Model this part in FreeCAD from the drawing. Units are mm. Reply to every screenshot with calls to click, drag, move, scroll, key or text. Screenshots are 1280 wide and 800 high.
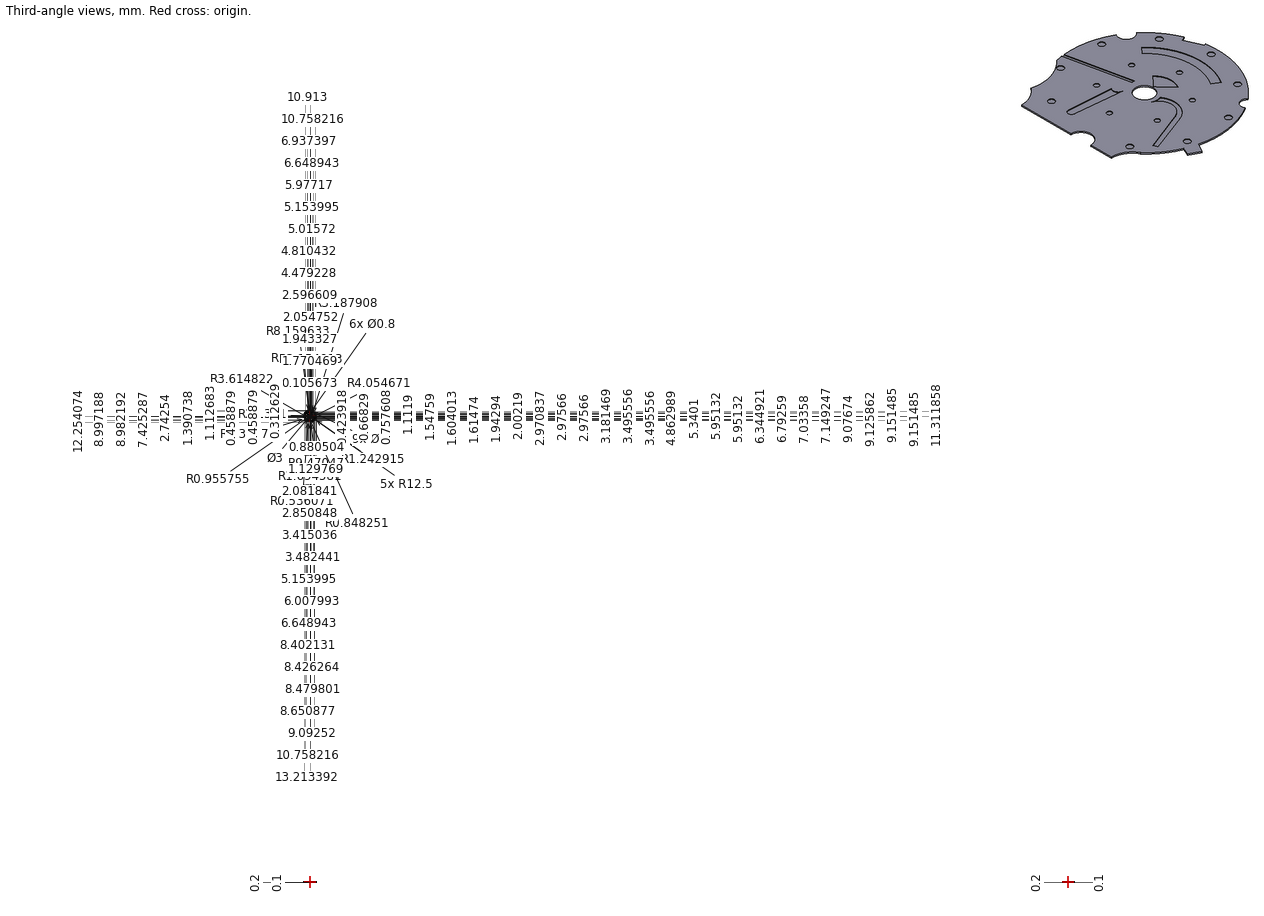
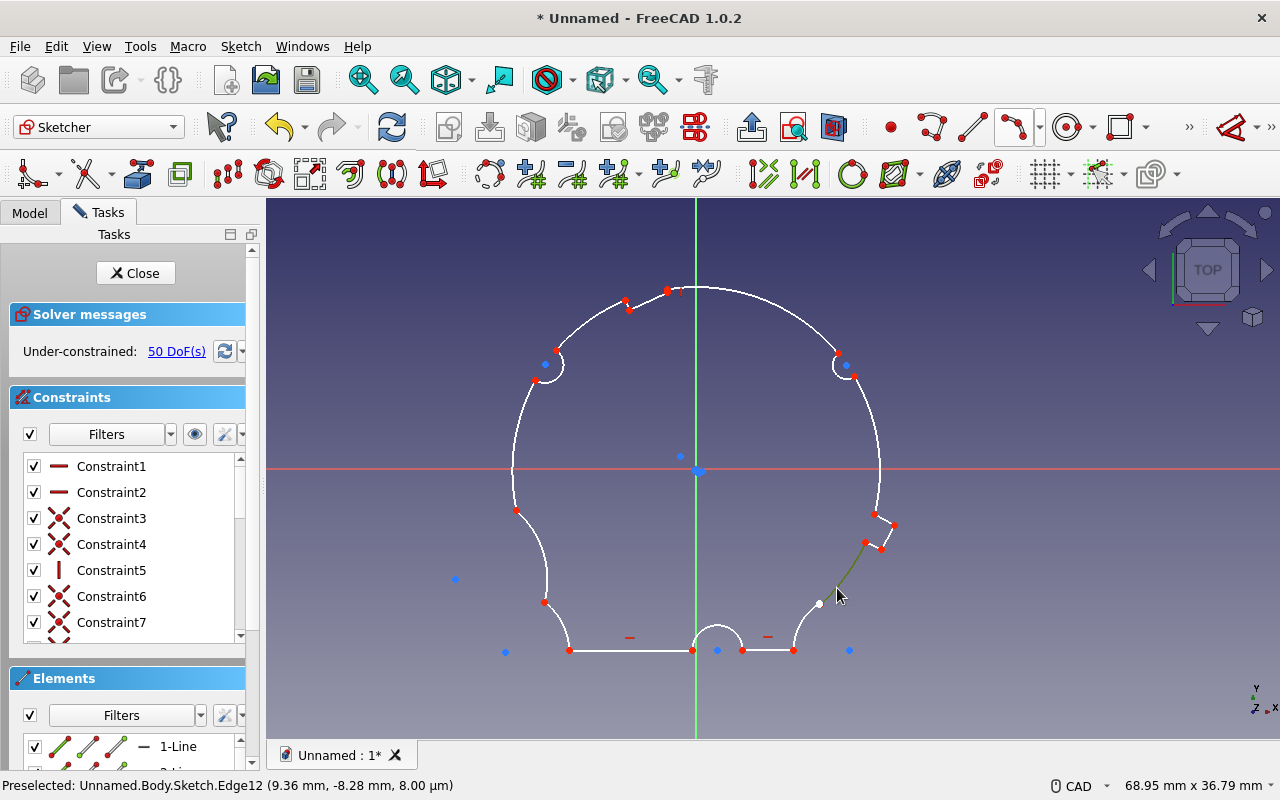
click(880, 472)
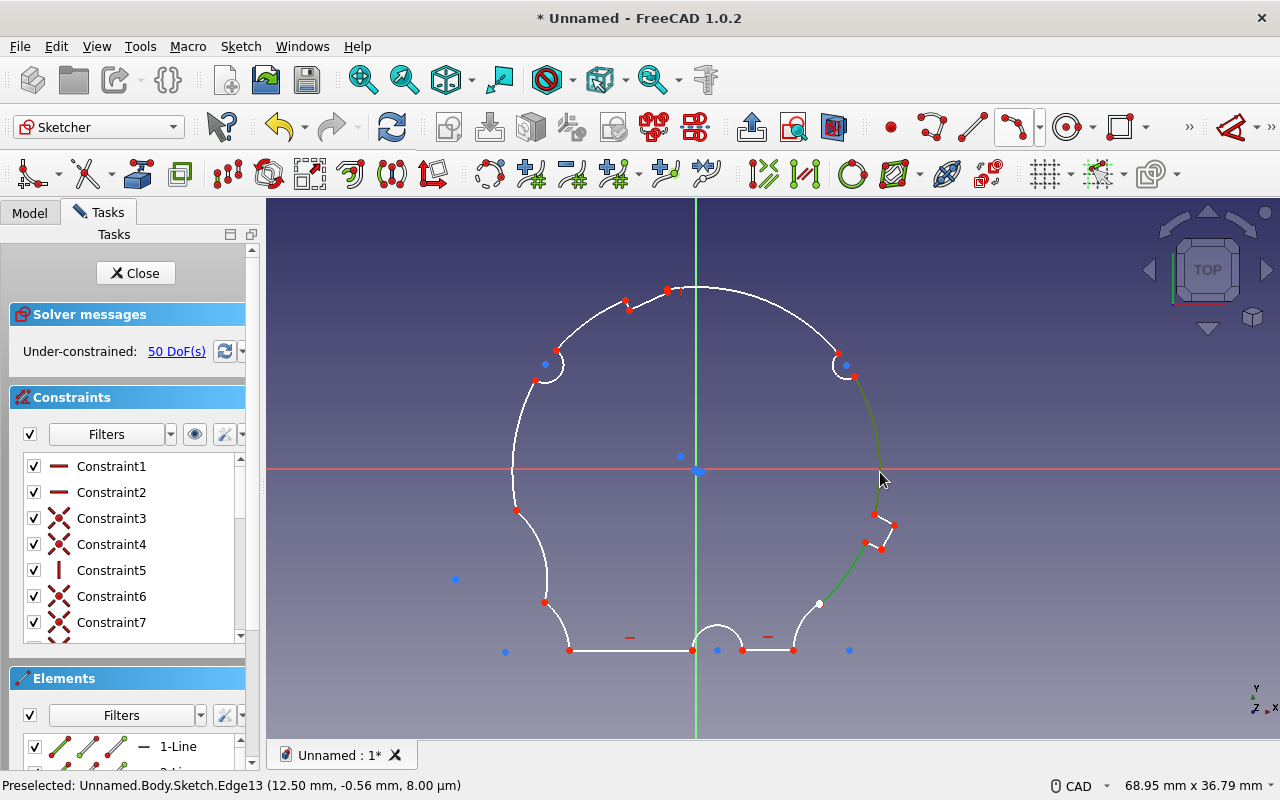
key(c)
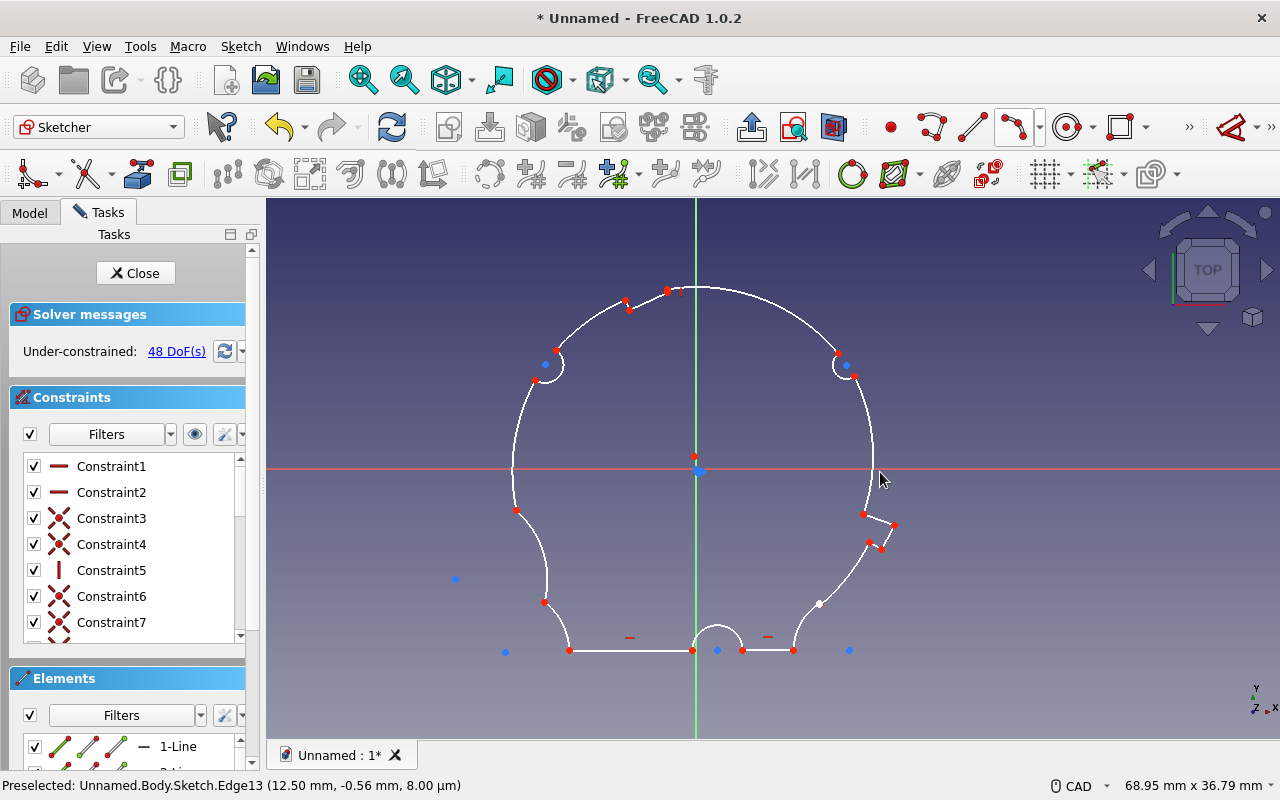
click(838, 588)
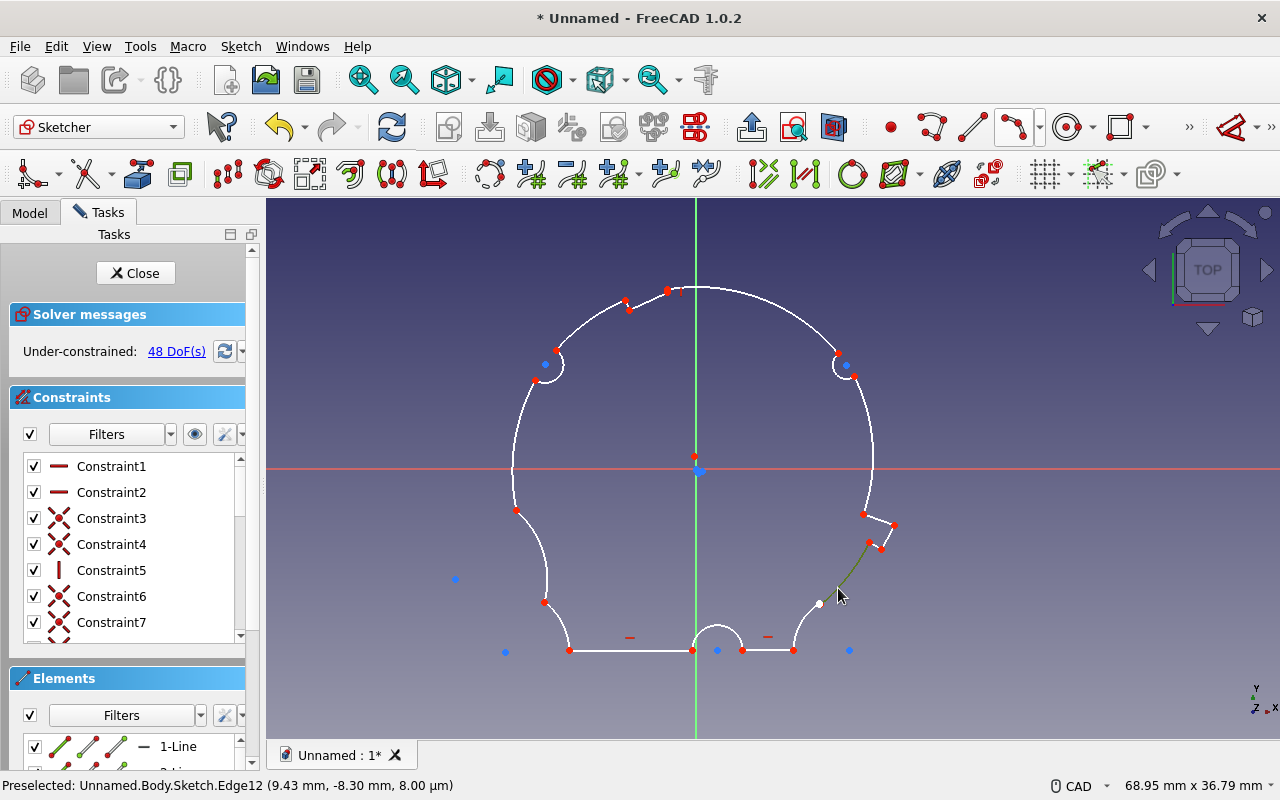
click(796, 316)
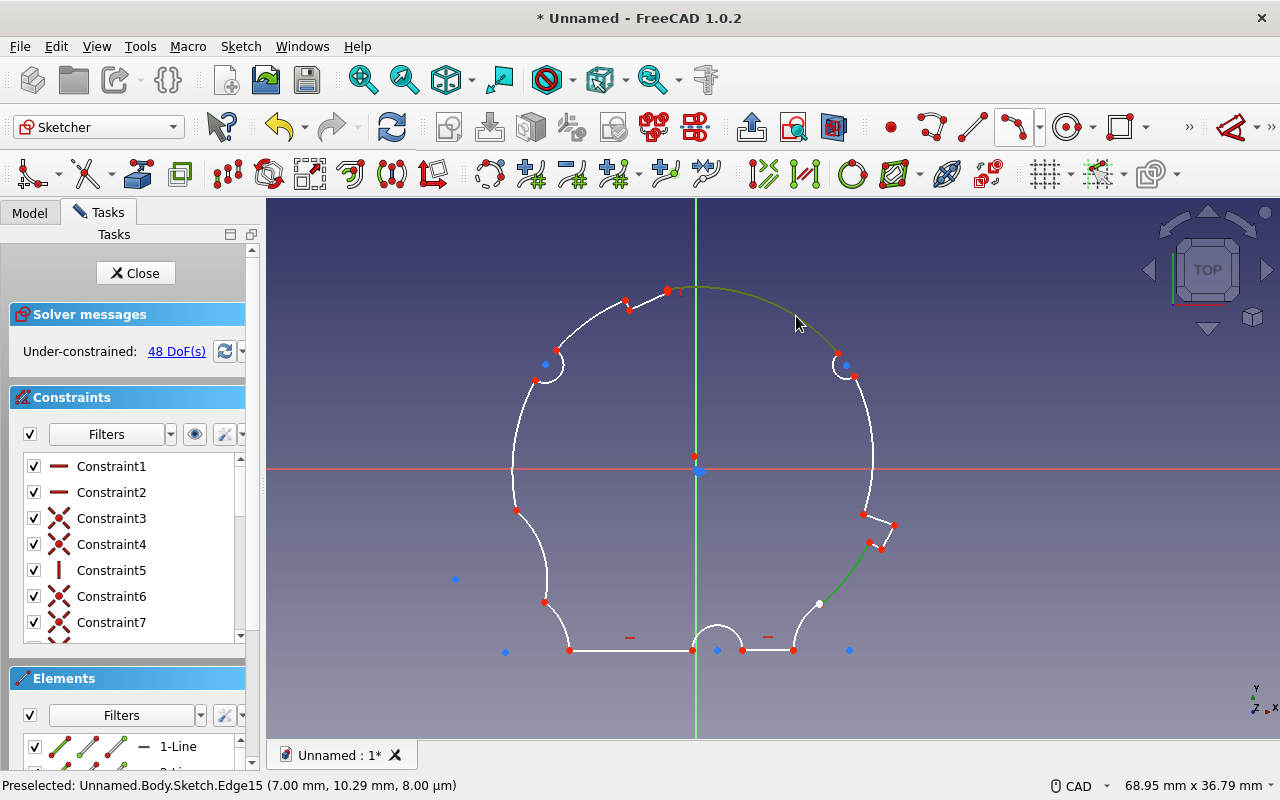
key(c)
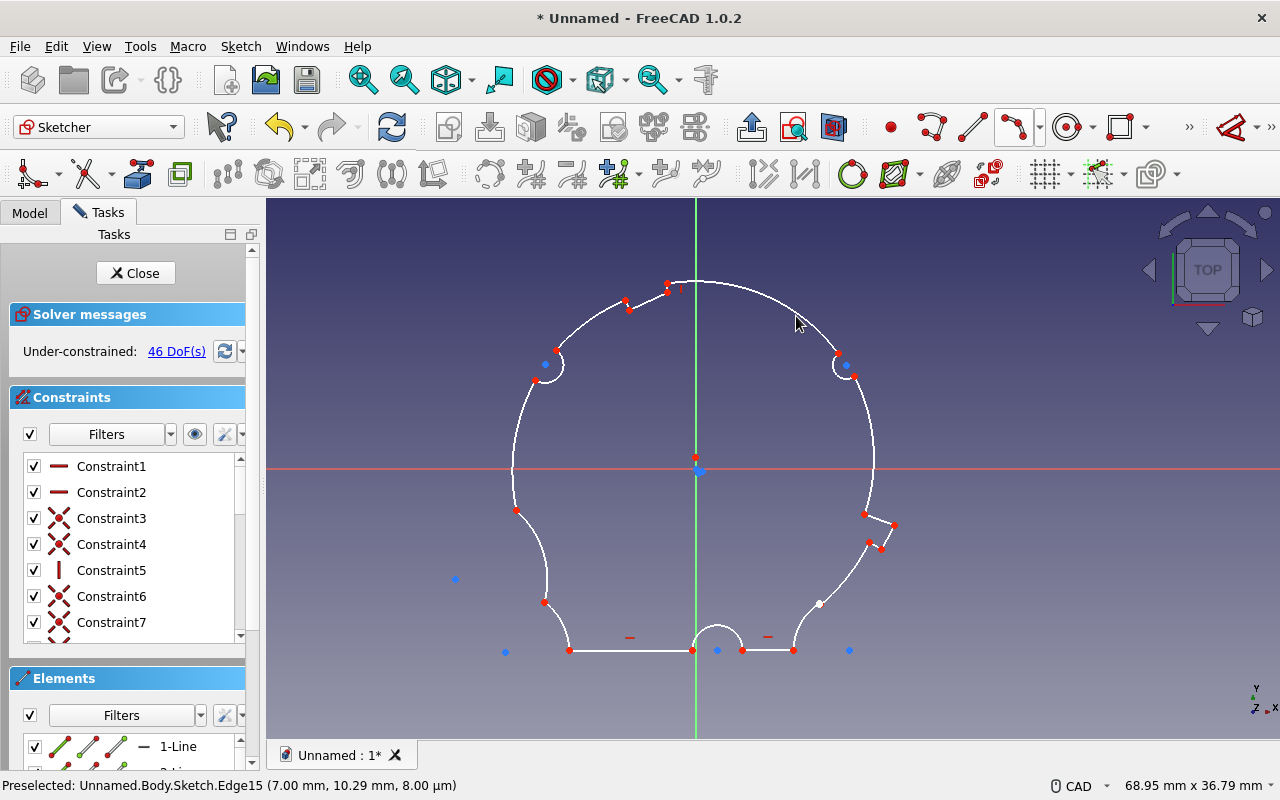
click(838, 588)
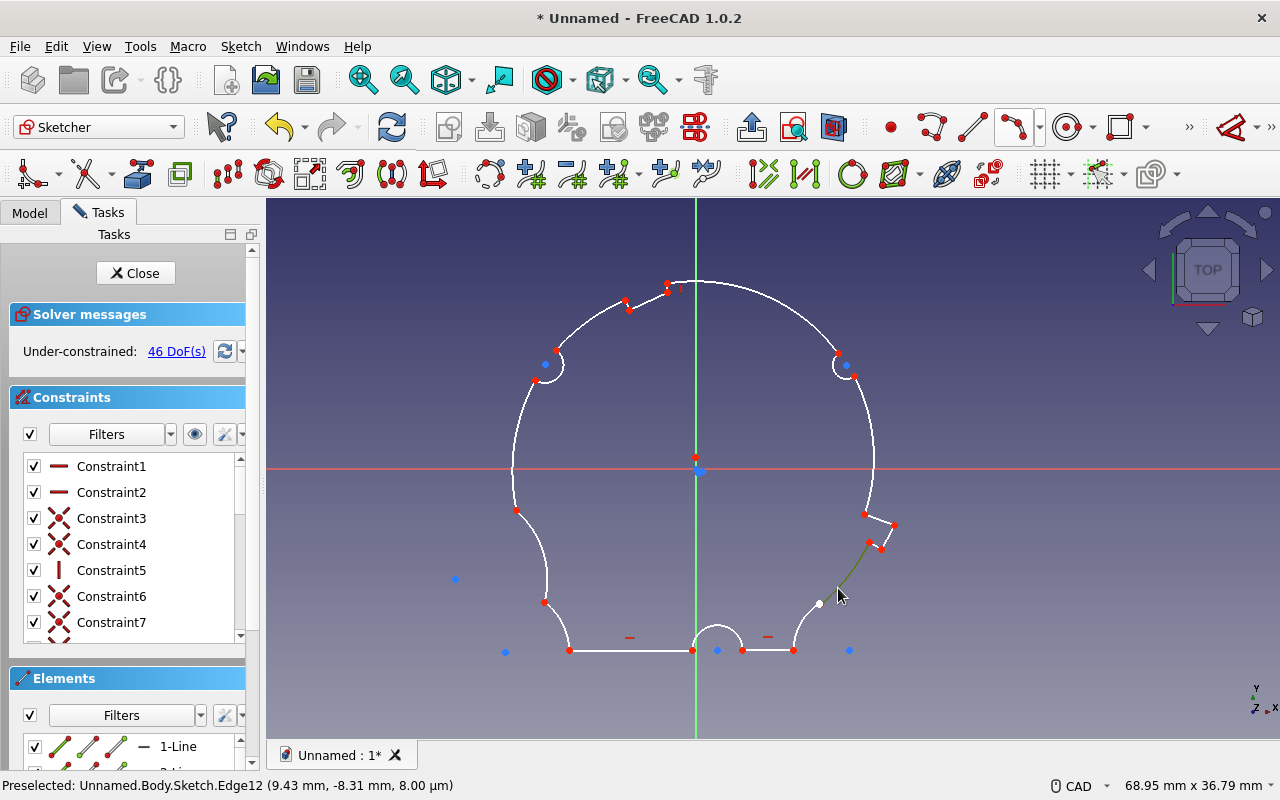
click(602, 312)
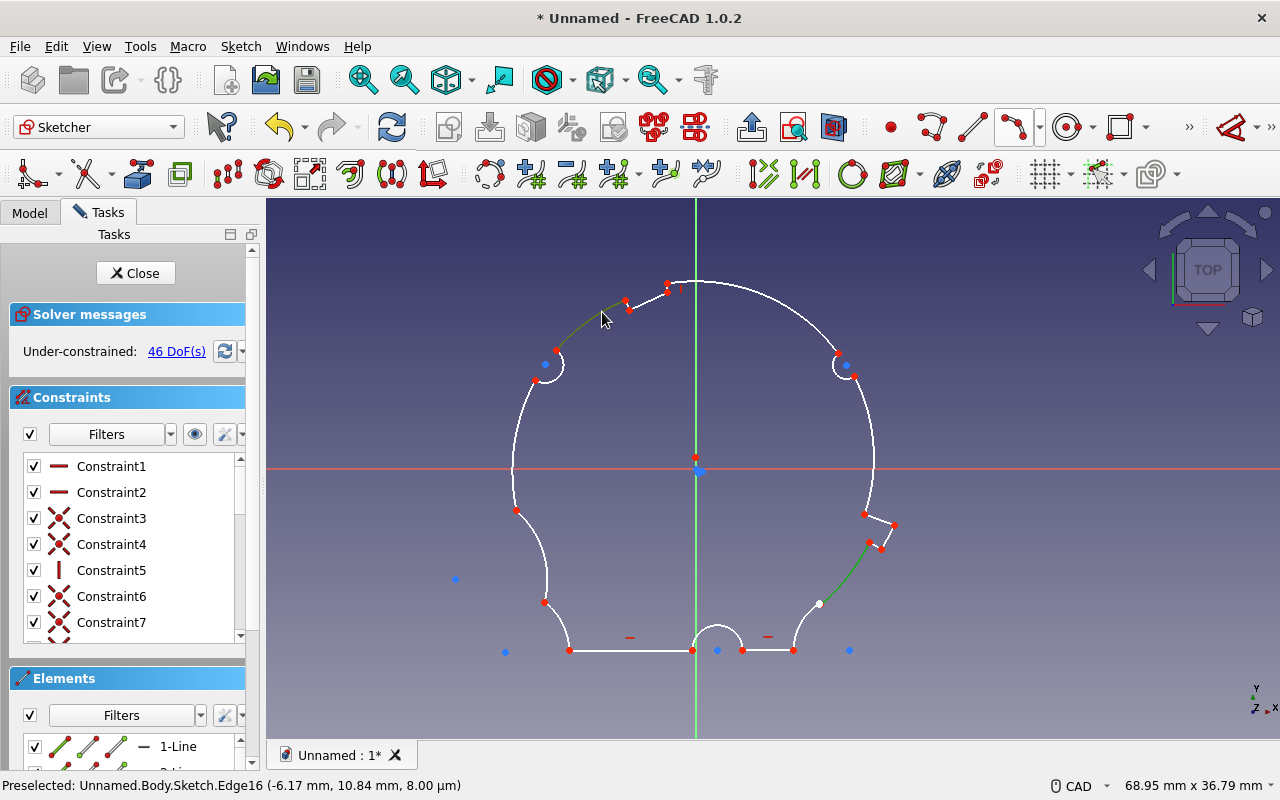
key(c)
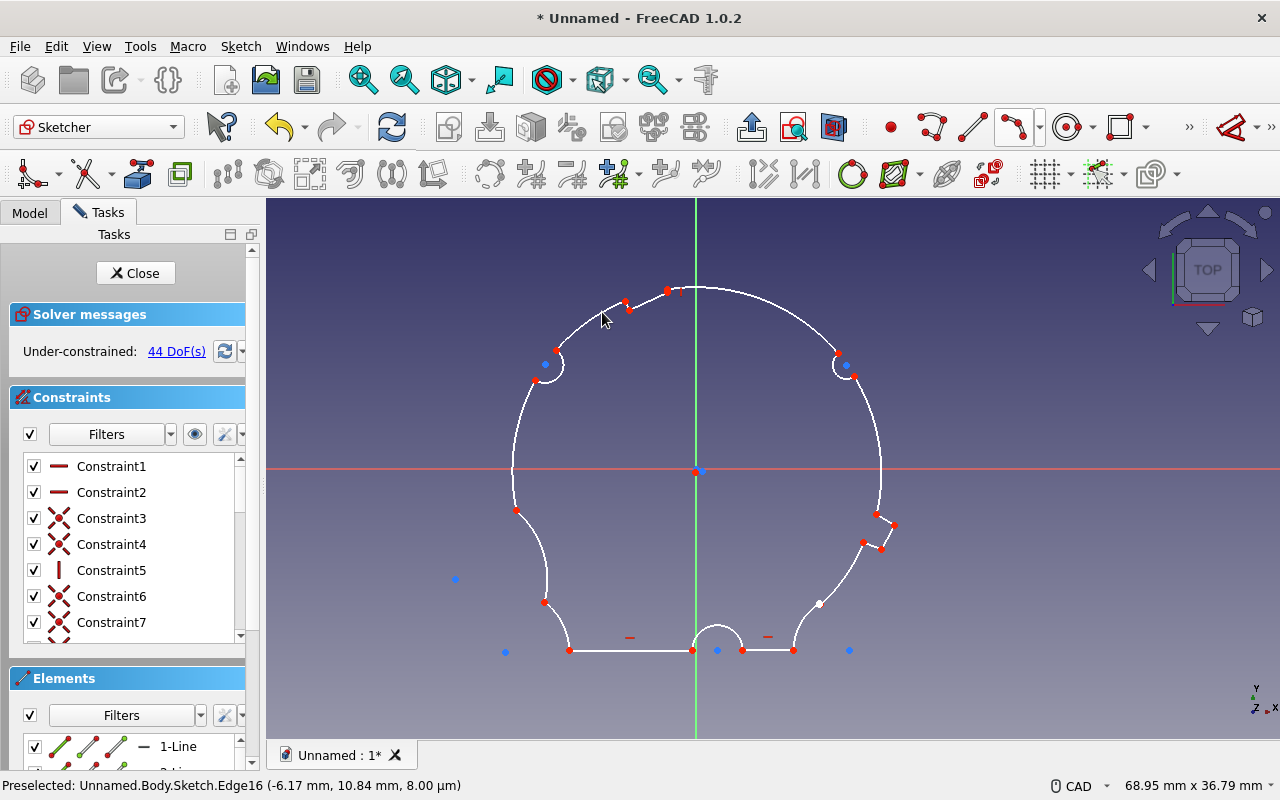
click(837, 588)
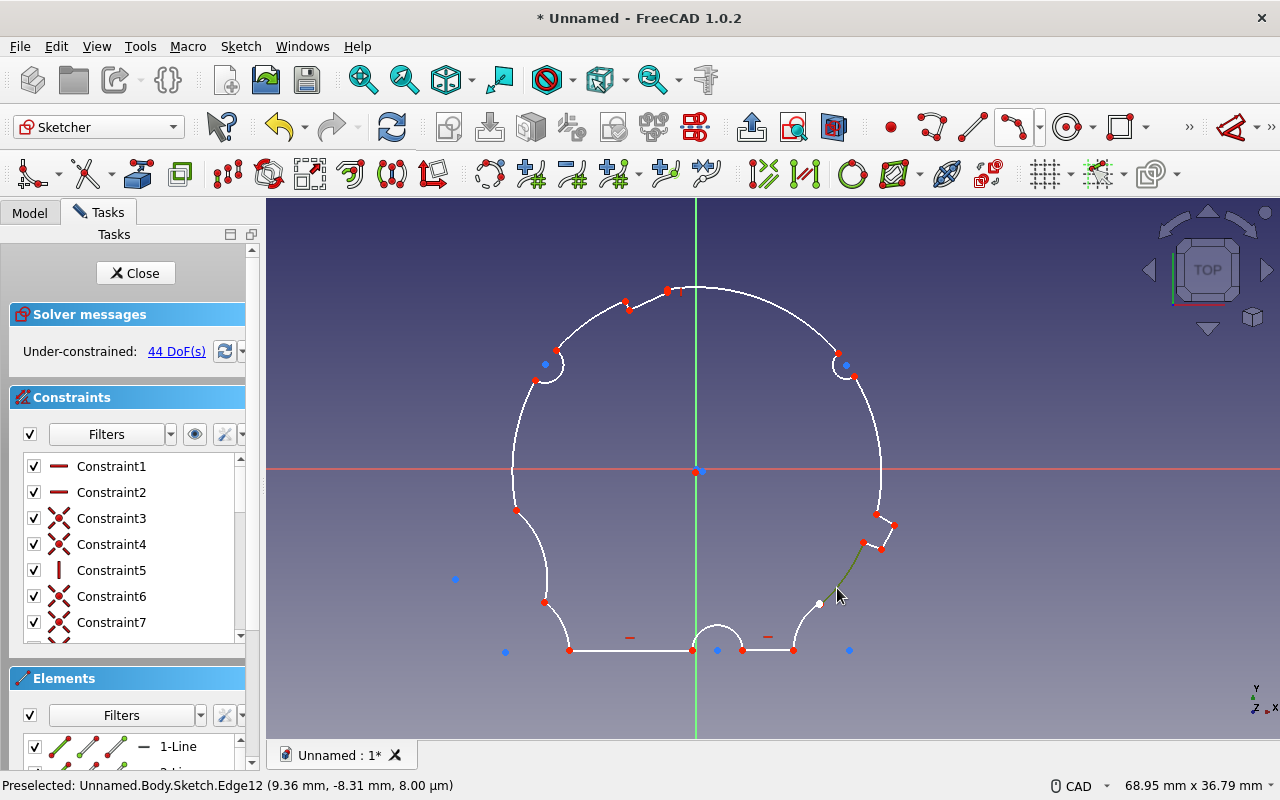
click(520, 418)